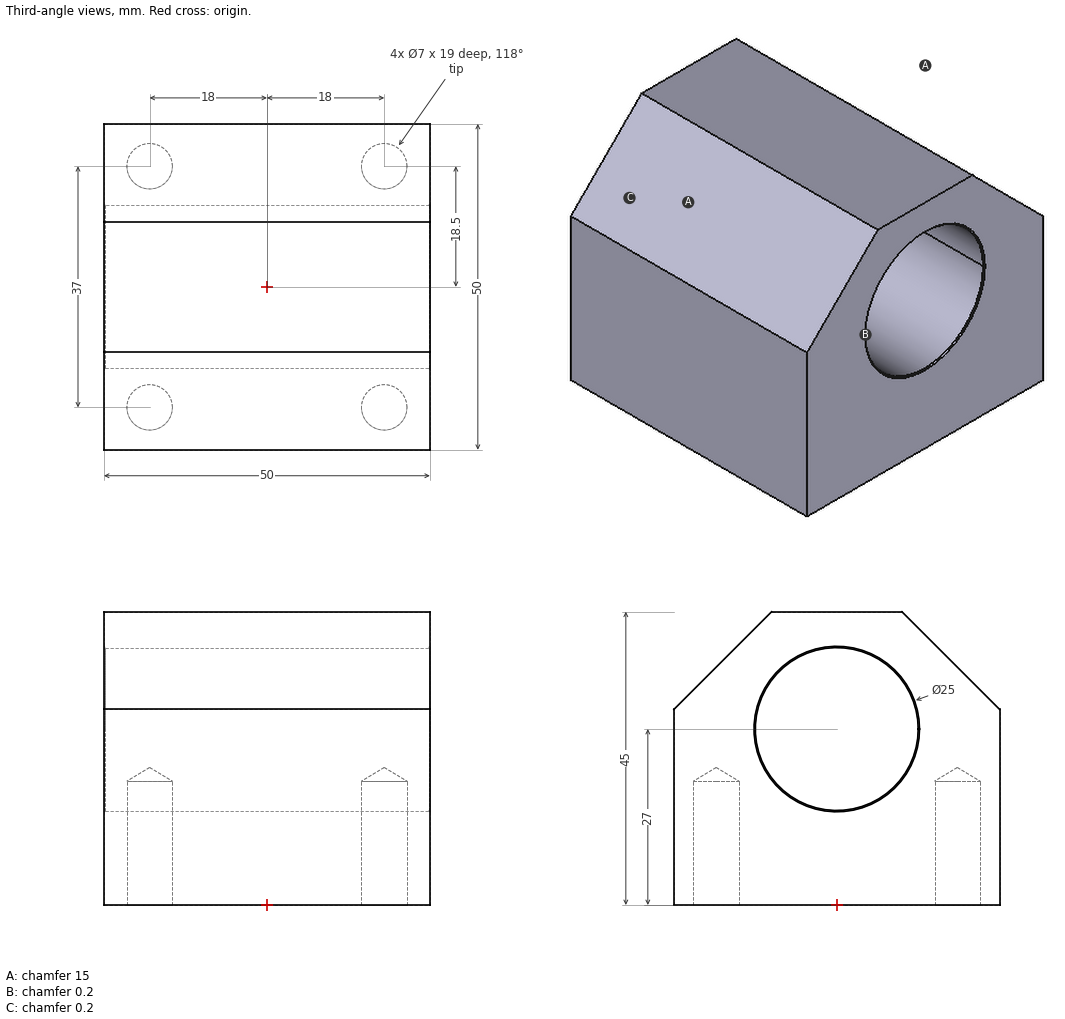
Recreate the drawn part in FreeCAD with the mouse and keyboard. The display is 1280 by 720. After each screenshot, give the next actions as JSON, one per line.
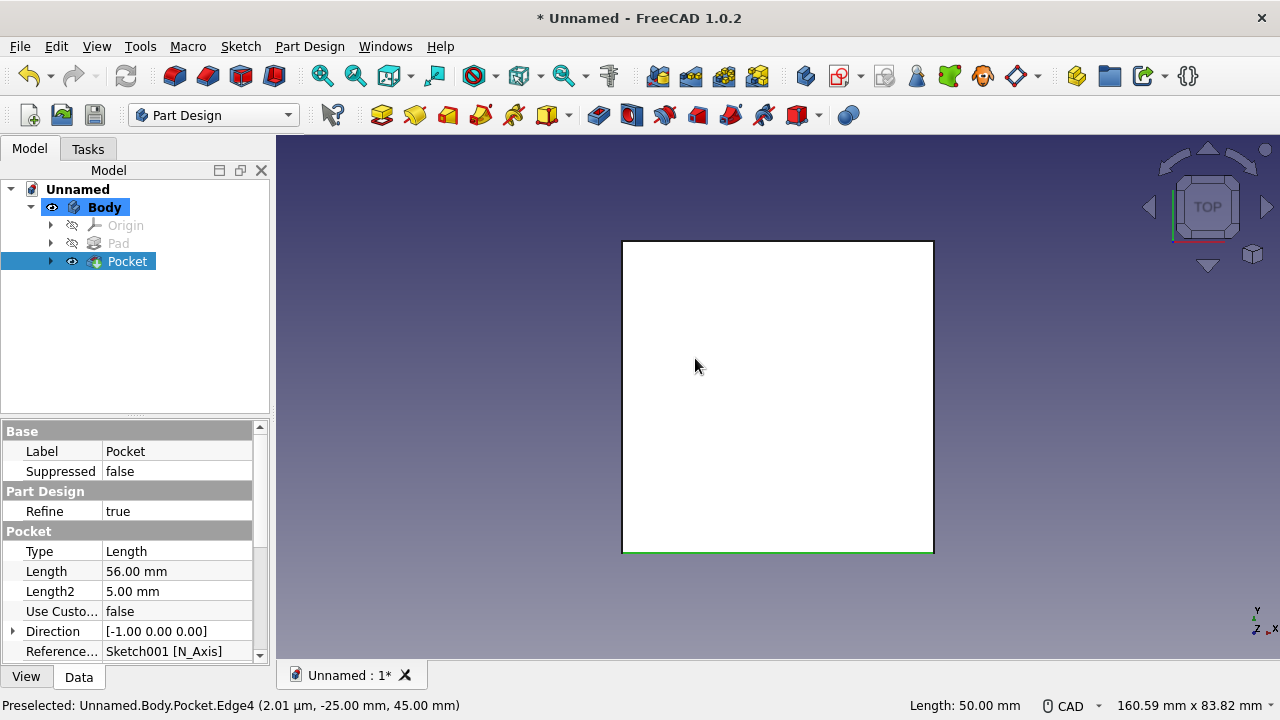
{"action": "left_click", "coordinate": [778, 240], "text": "ctrl"}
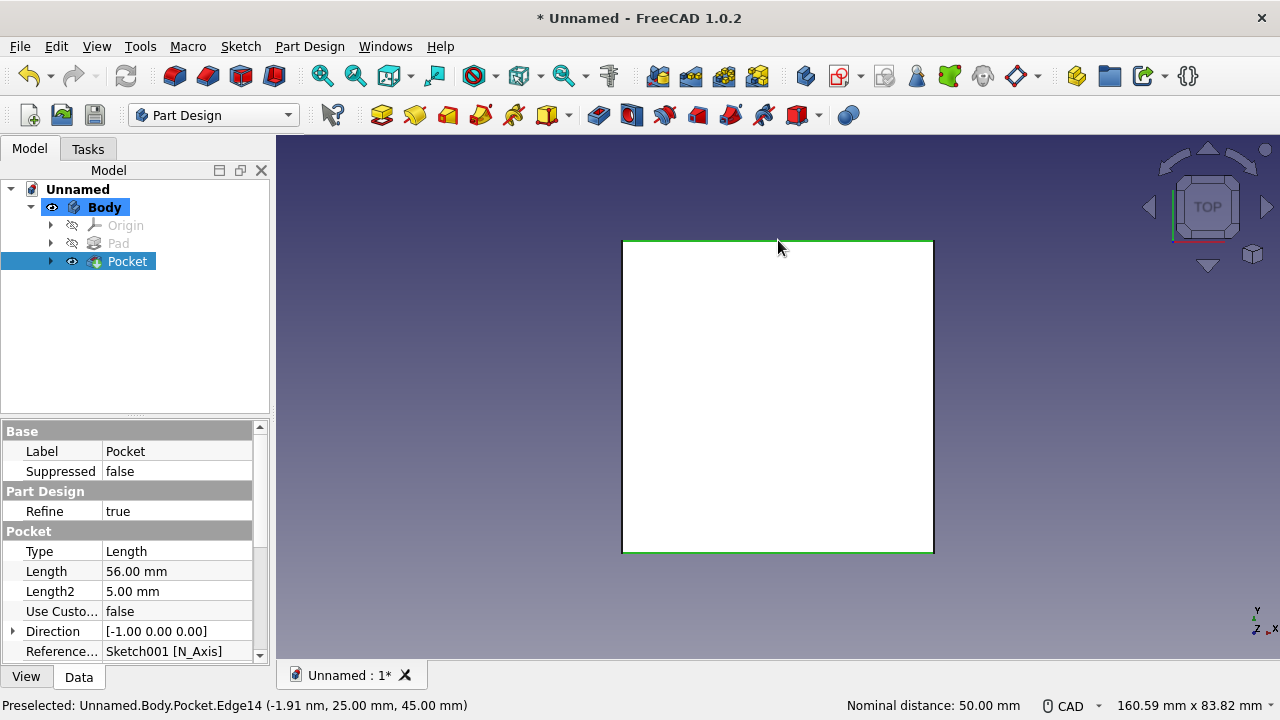
{"action": "left_click", "coordinate": [208, 76]}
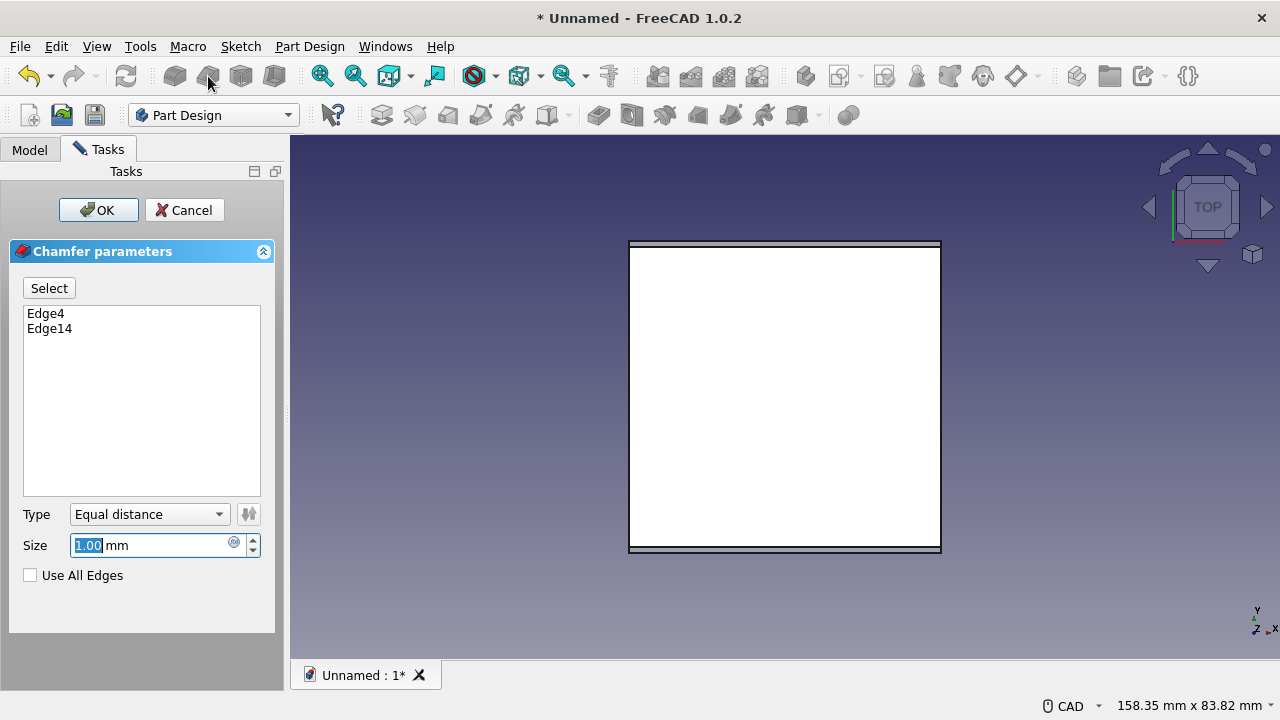
{"action": "type", "text": "15"}
{"action": "key", "text": "Tab"}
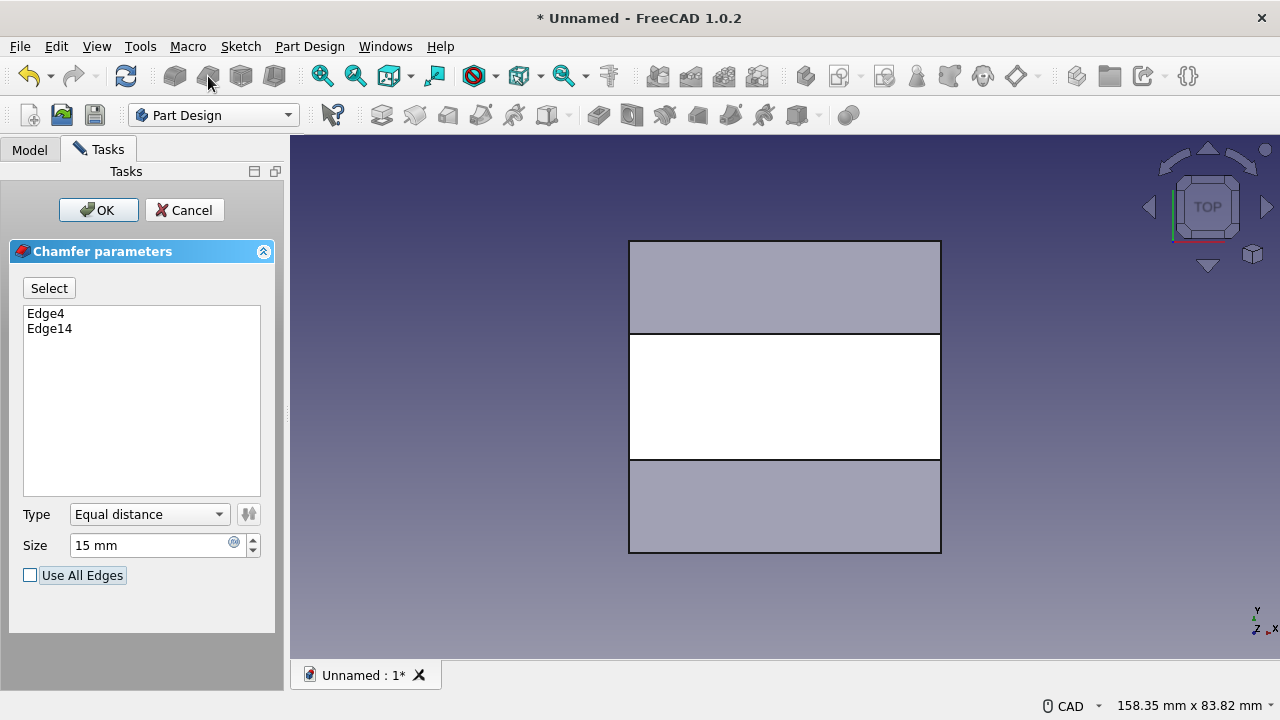
{"action": "left_click", "coordinate": [99, 210]}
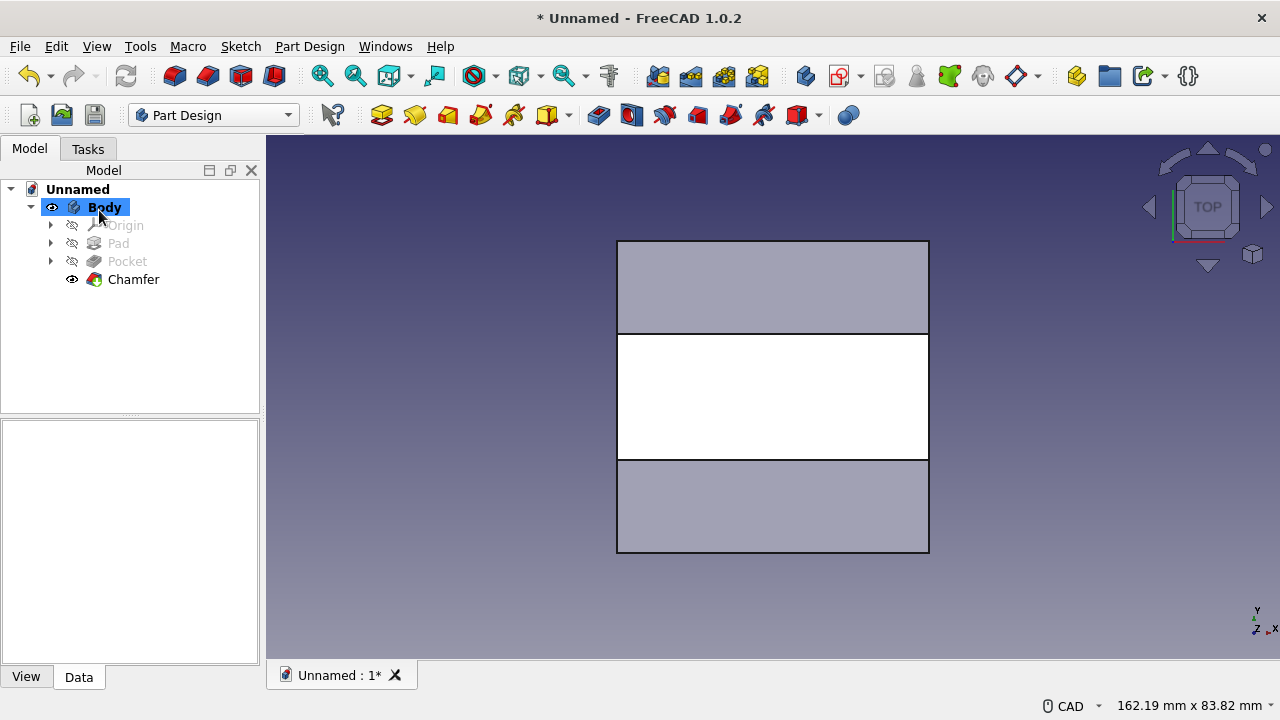
{"action": "left_click", "coordinate": [838, 76]}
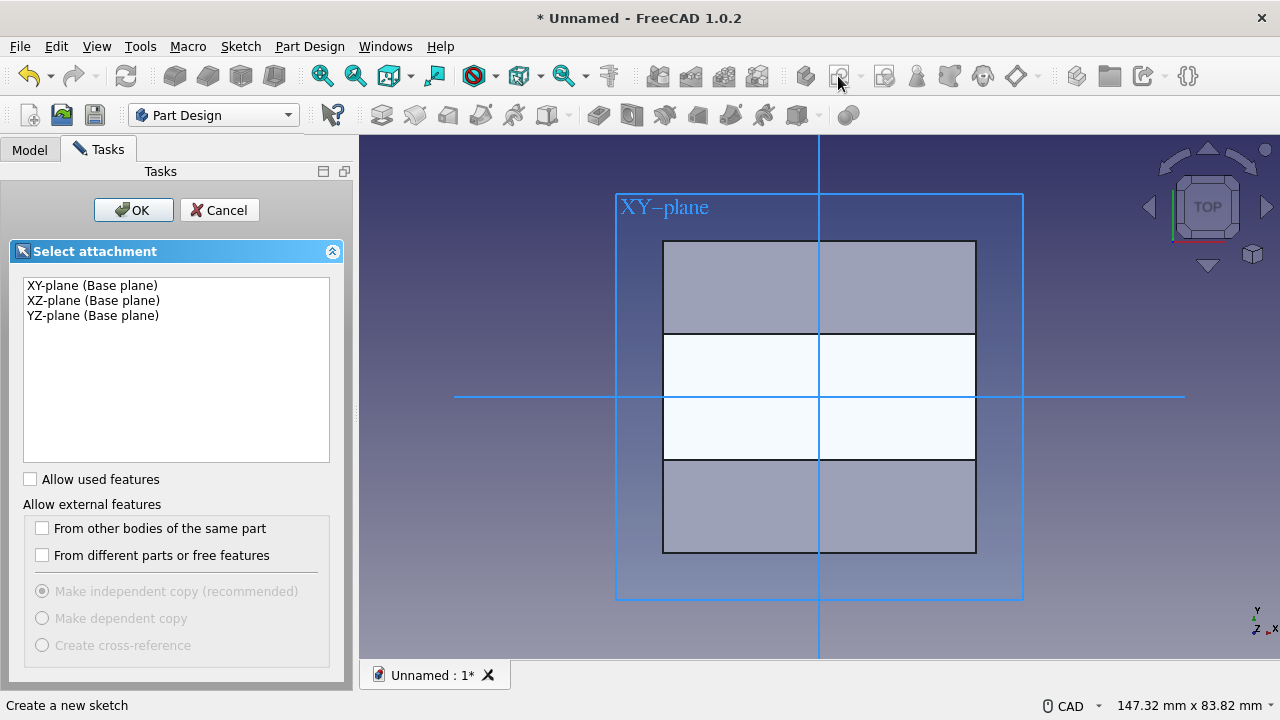
{"action": "left_click", "coordinate": [84, 286]}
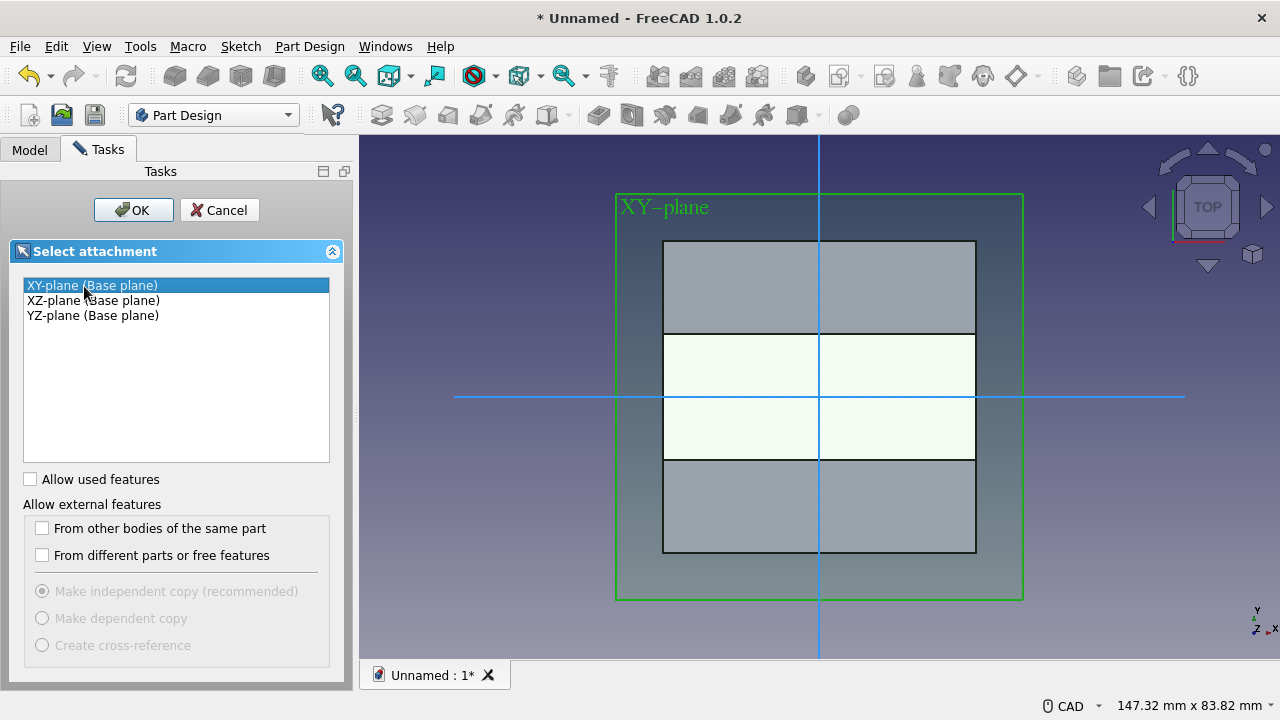
{"action": "left_click", "coordinate": [134, 210]}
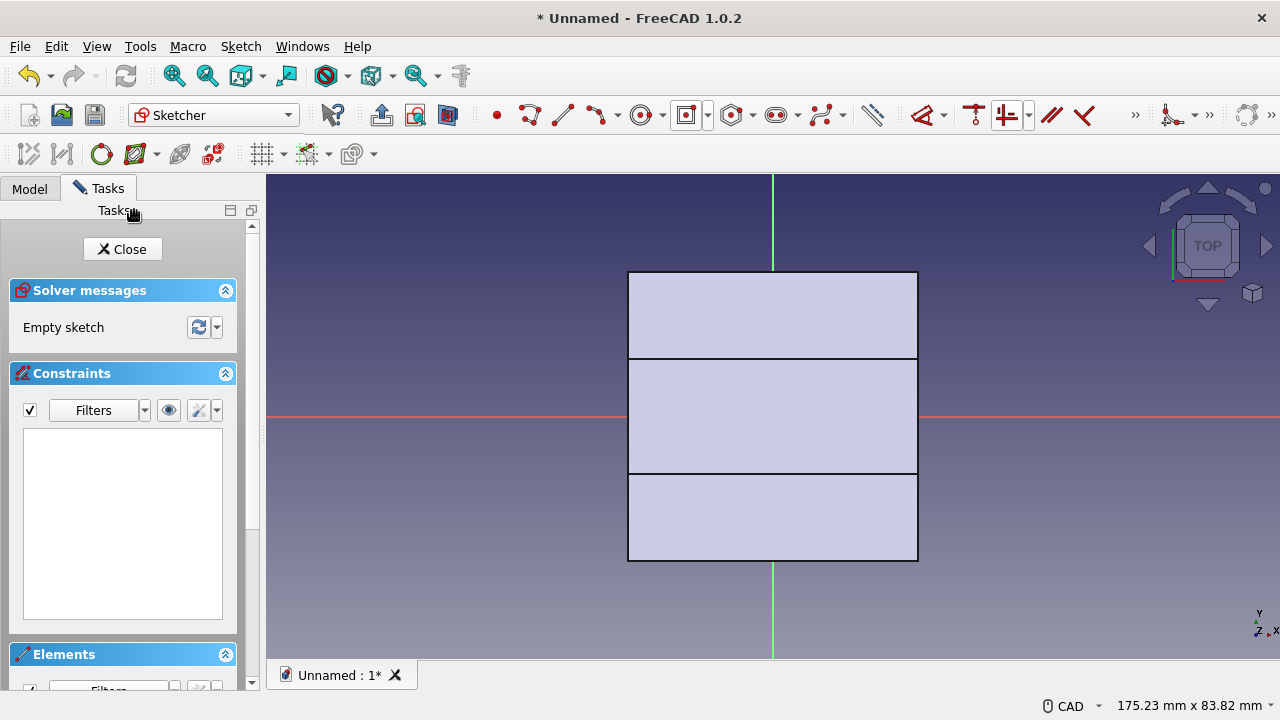
{"action": "left_click", "coordinate": [448, 116]}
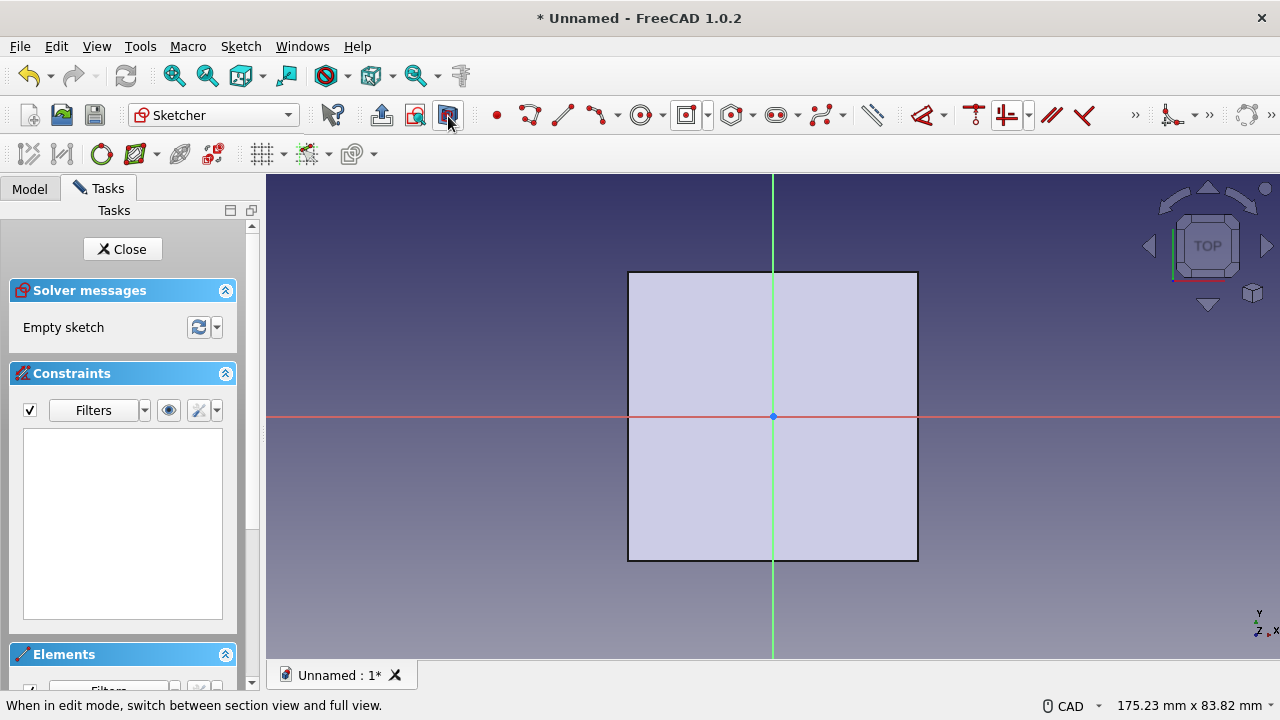
{"action": "left_click", "coordinate": [640, 116]}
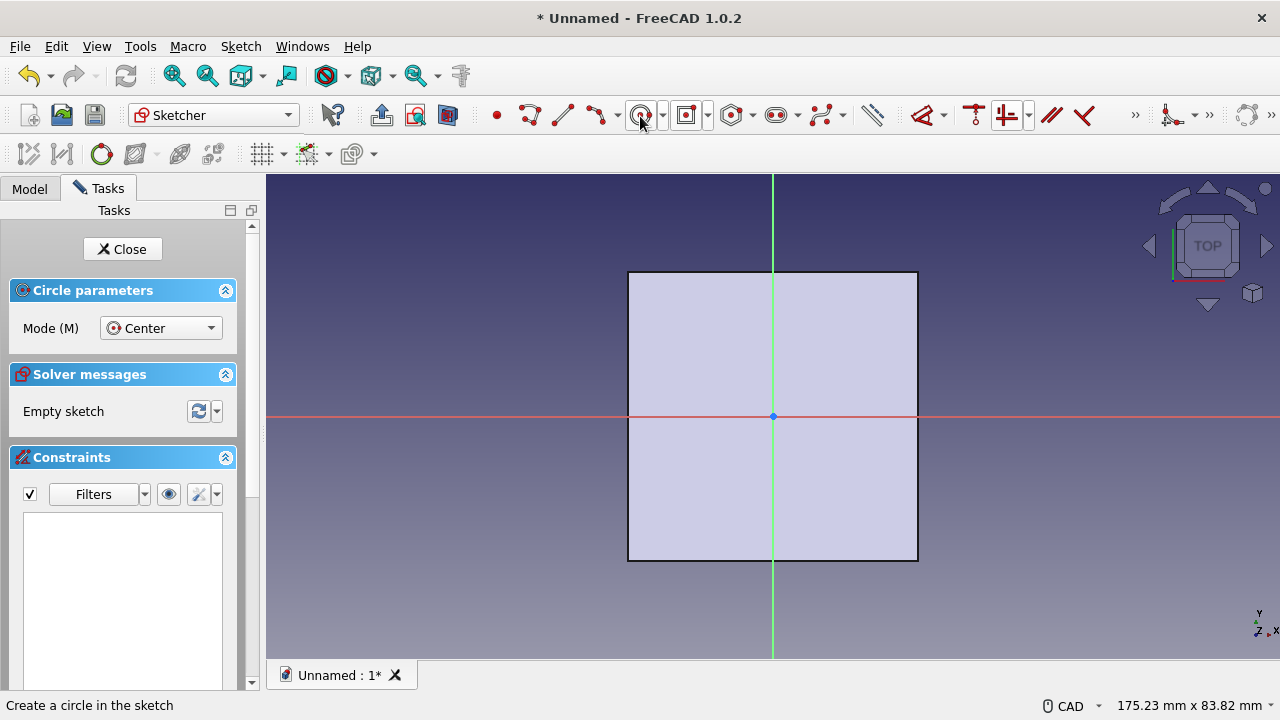
{"action": "left_click", "coordinate": [877, 309]}
{"action": "left_click", "coordinate": [891, 295]}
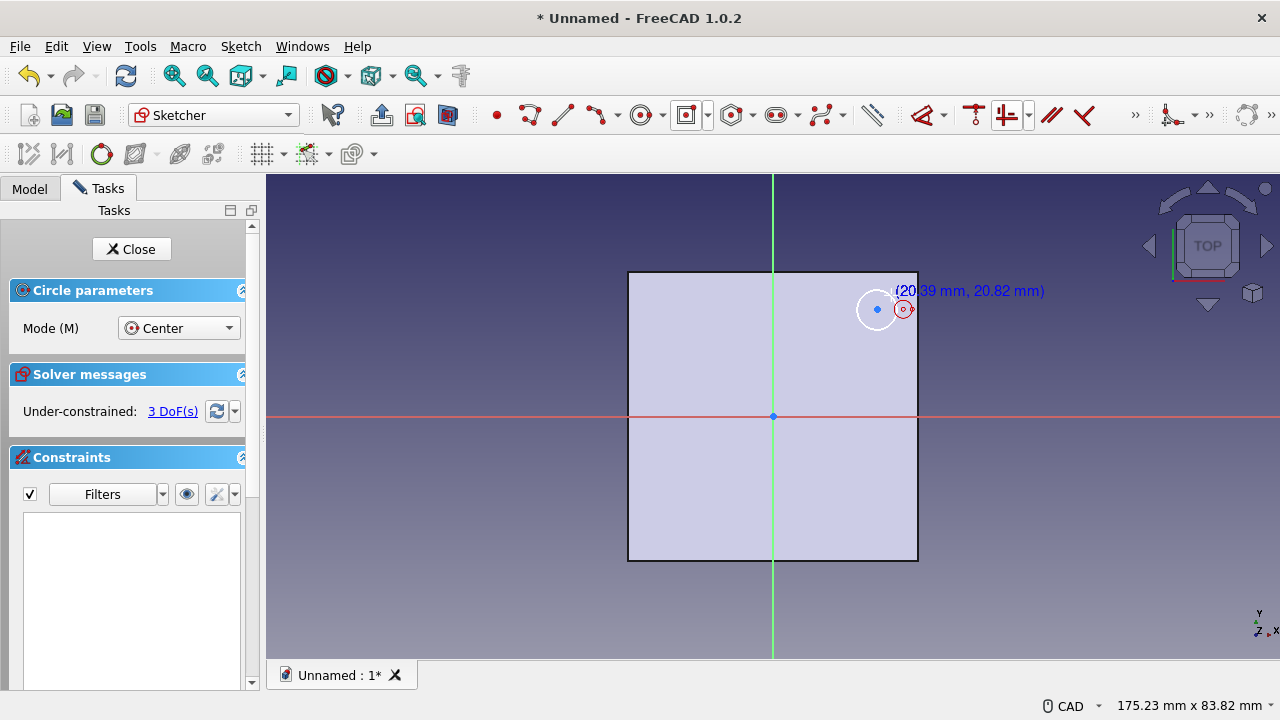
{"action": "left_click", "coordinate": [669, 309]}
{"action": "left_click", "coordinate": [683, 295]}